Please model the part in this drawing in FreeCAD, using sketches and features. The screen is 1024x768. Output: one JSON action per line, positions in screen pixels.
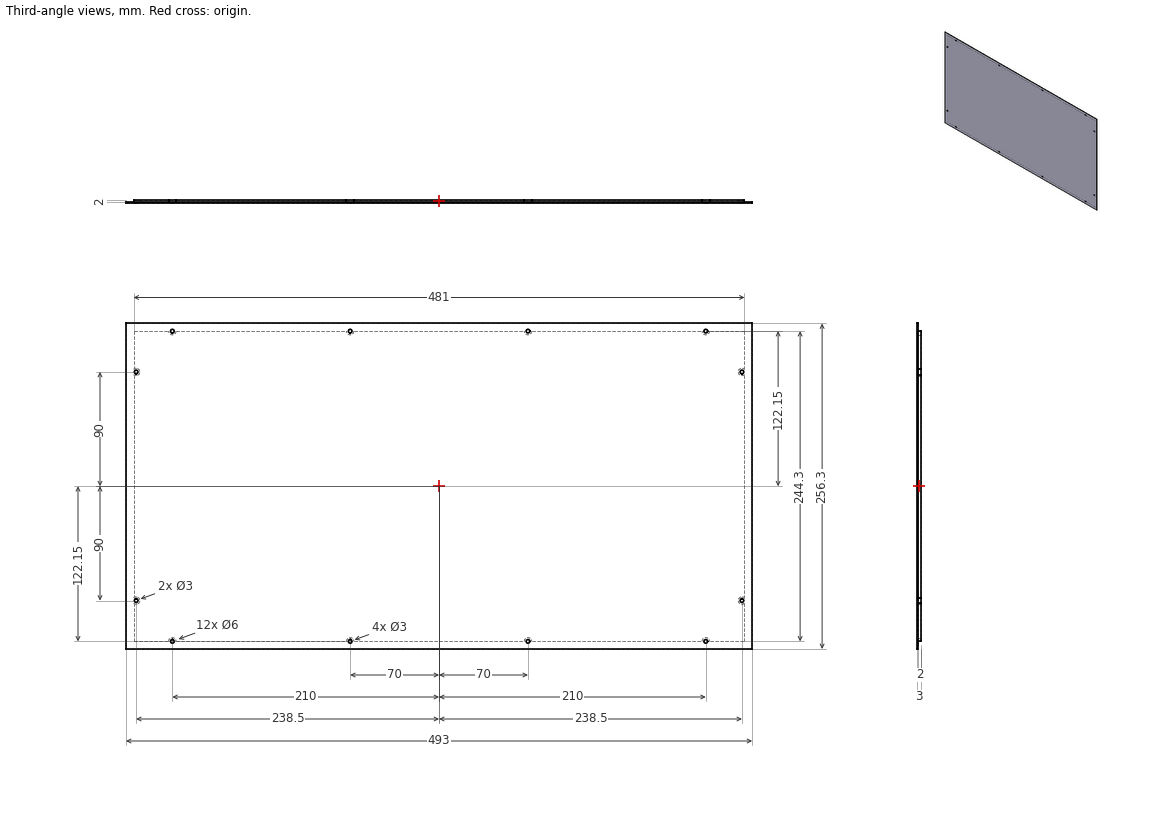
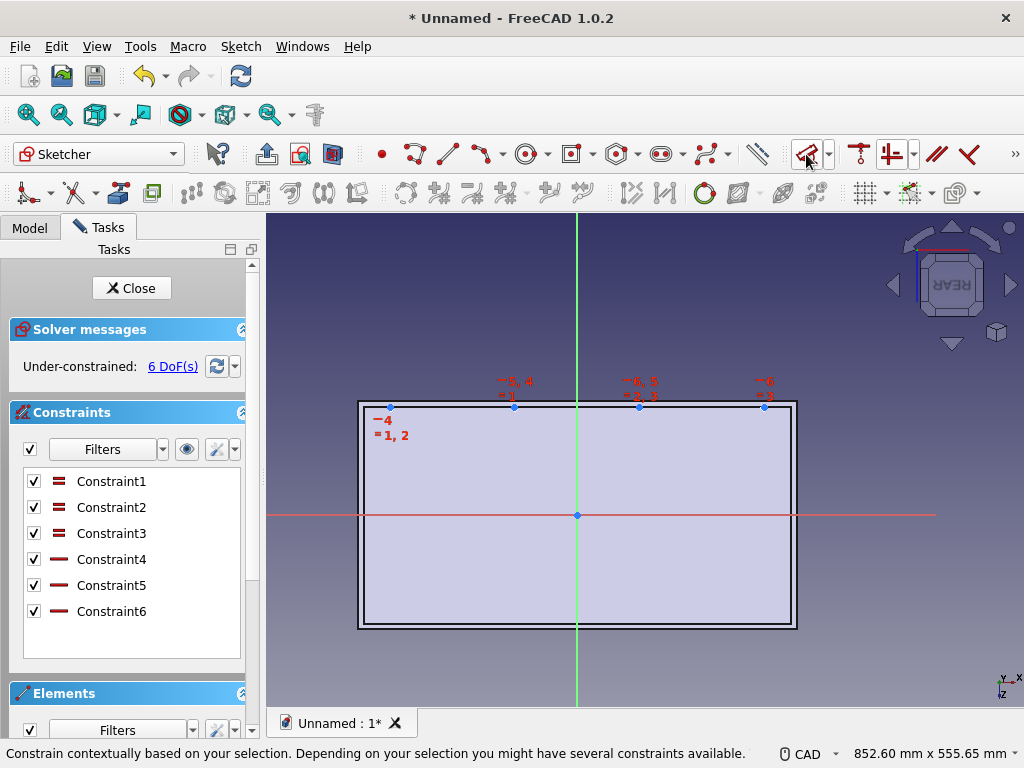
{"action": "scroll", "coordinate": [517, 406], "scroll_direction": "up", "scroll_amount": 14}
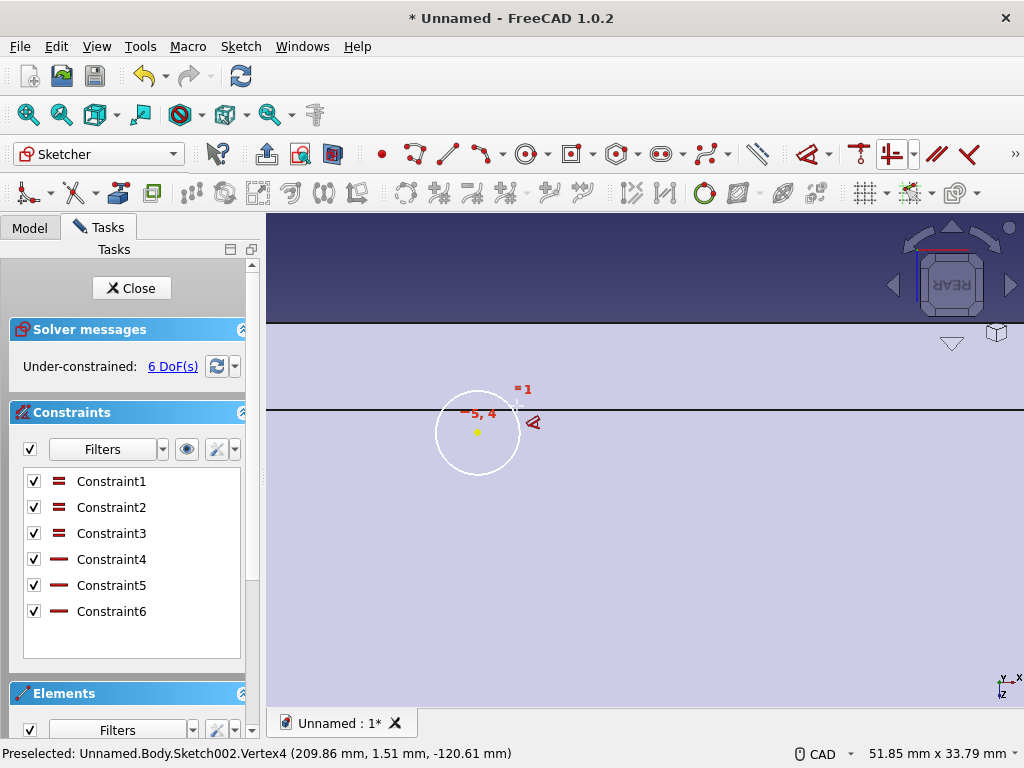
{"action": "left_click", "coordinate": [507, 403]}
{"action": "left_click", "coordinate": [529, 380]}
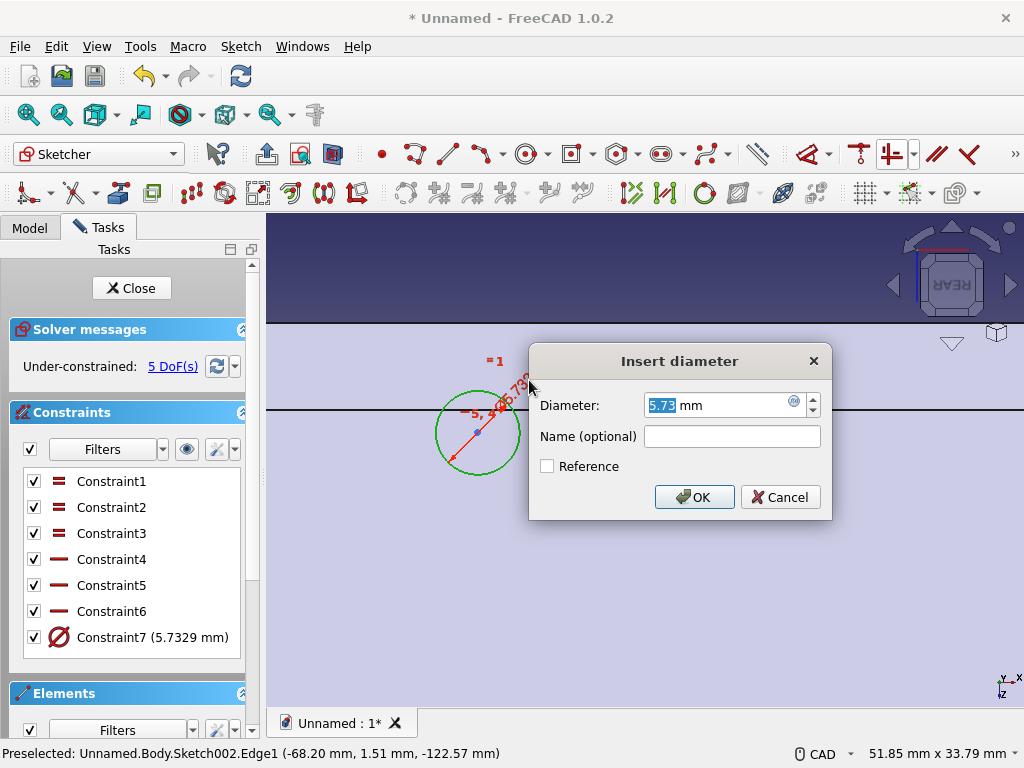
{"action": "type", "text": "3"}
{"action": "key", "text": "Return"}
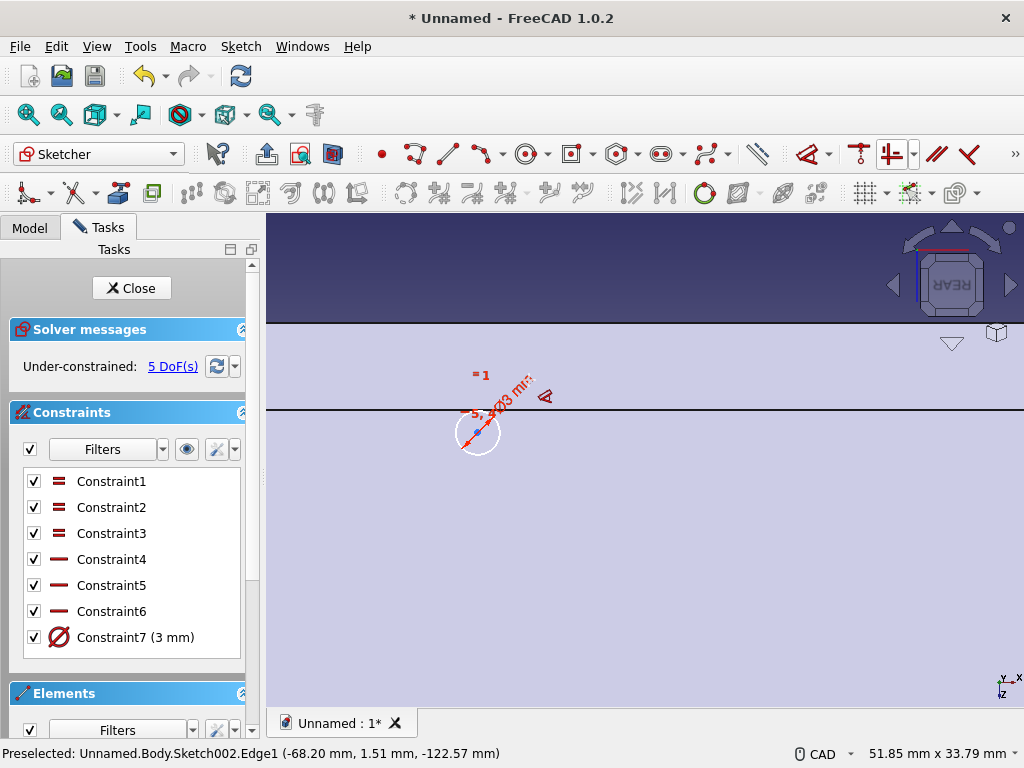
{"action": "scroll", "coordinate": [516, 406], "scroll_direction": "down", "scroll_amount": 14}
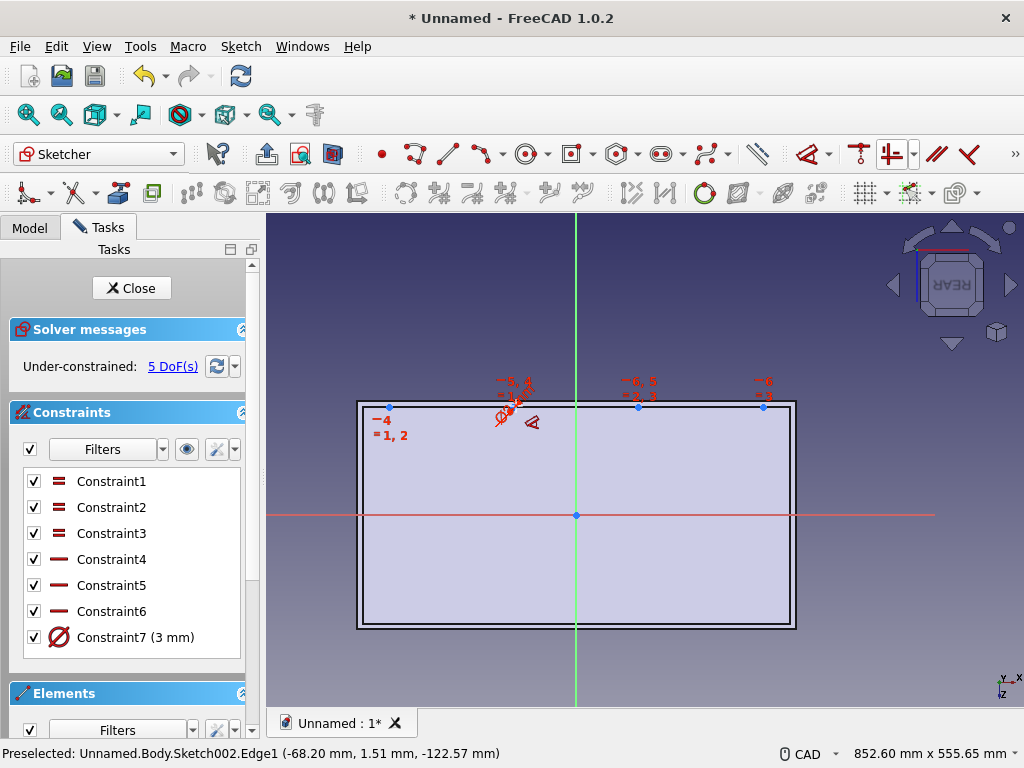
{"action": "left_click", "coordinate": [514, 408]}
{"action": "left_click", "coordinate": [545, 549]}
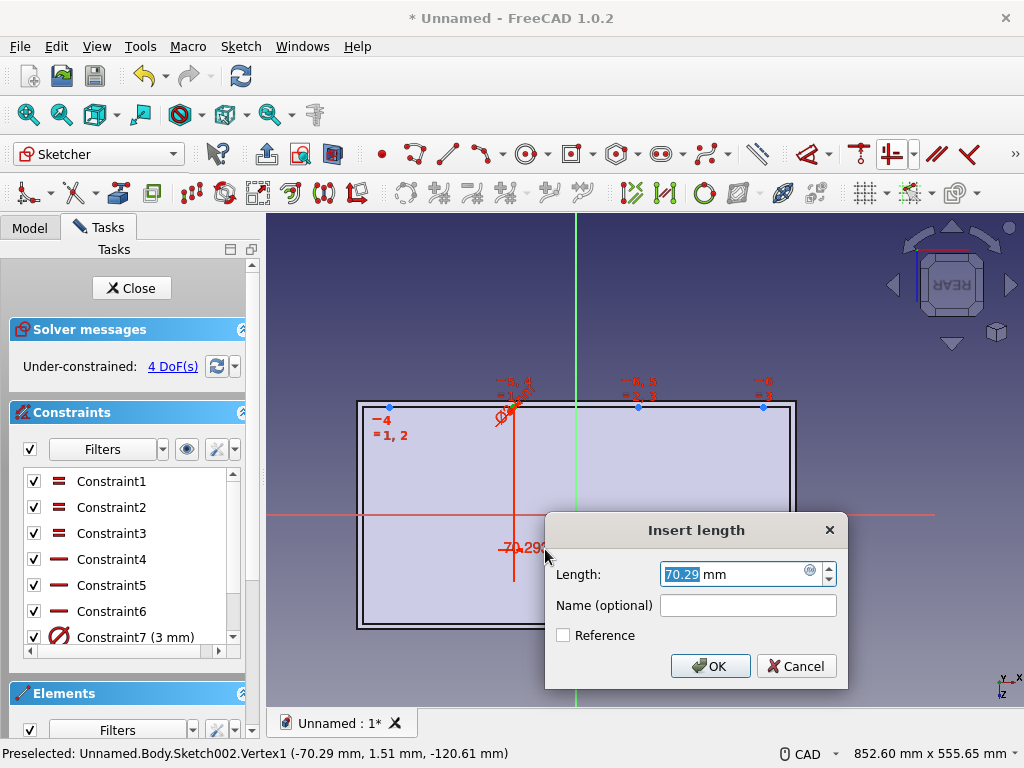
{"action": "type", "text": "70"}
{"action": "key", "text": "Return"}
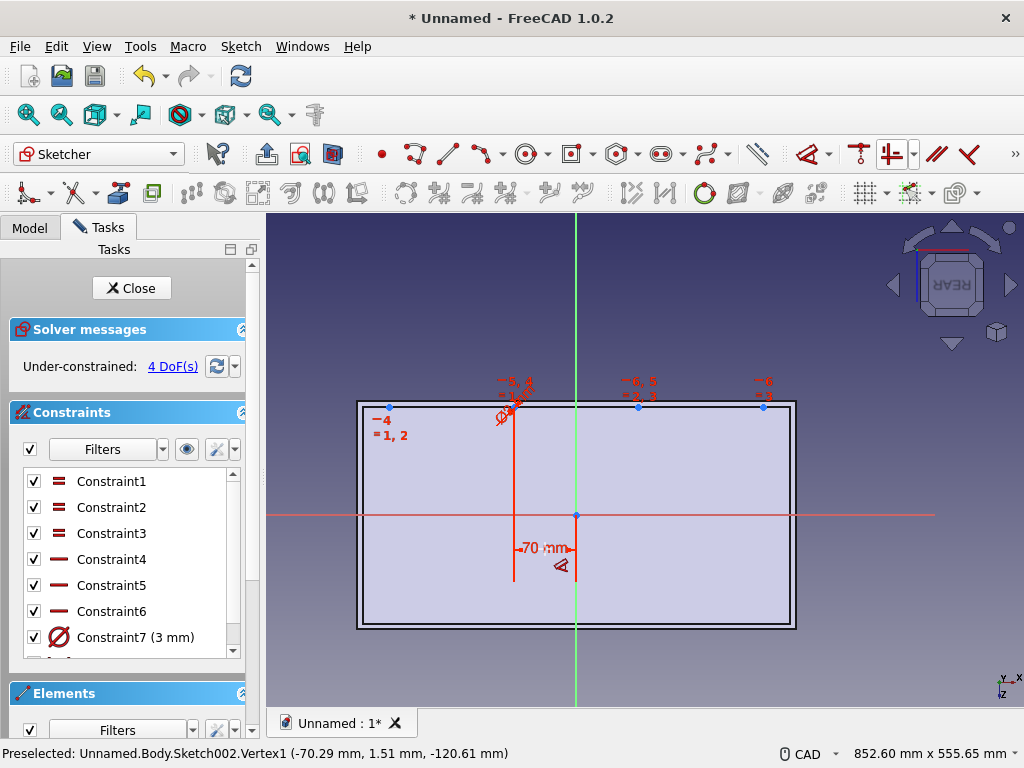
{"action": "left_click", "coordinate": [639, 408]}
{"action": "left_click", "coordinate": [622, 549]}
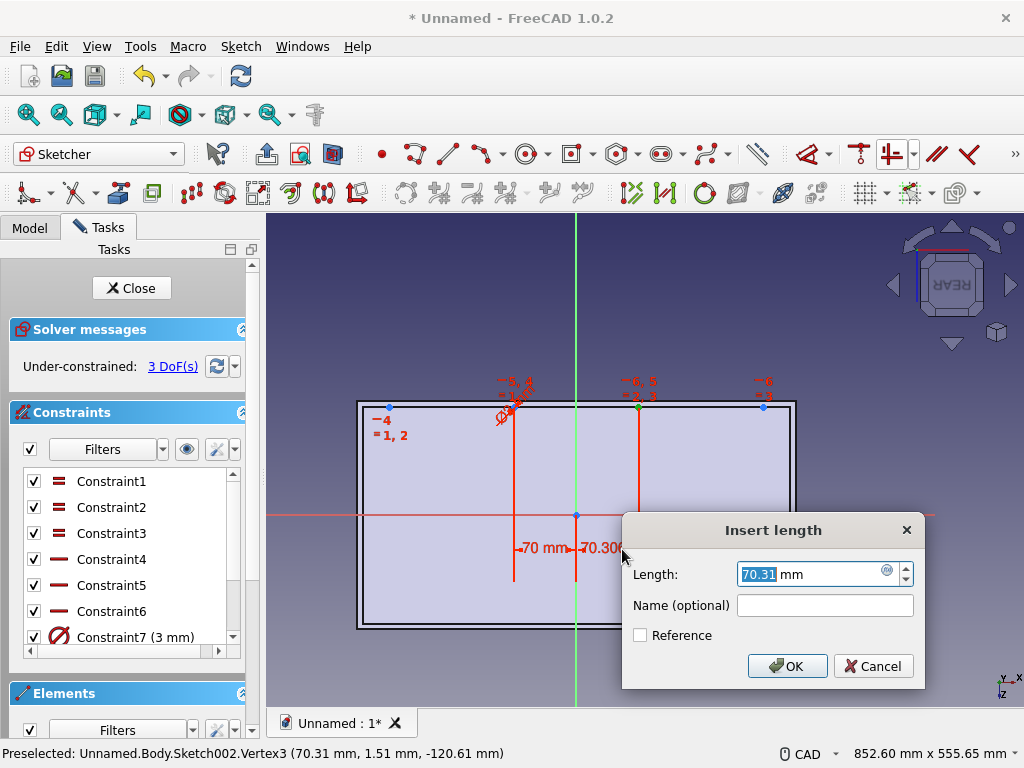
{"action": "type", "text": "70"}
{"action": "key", "text": "Return"}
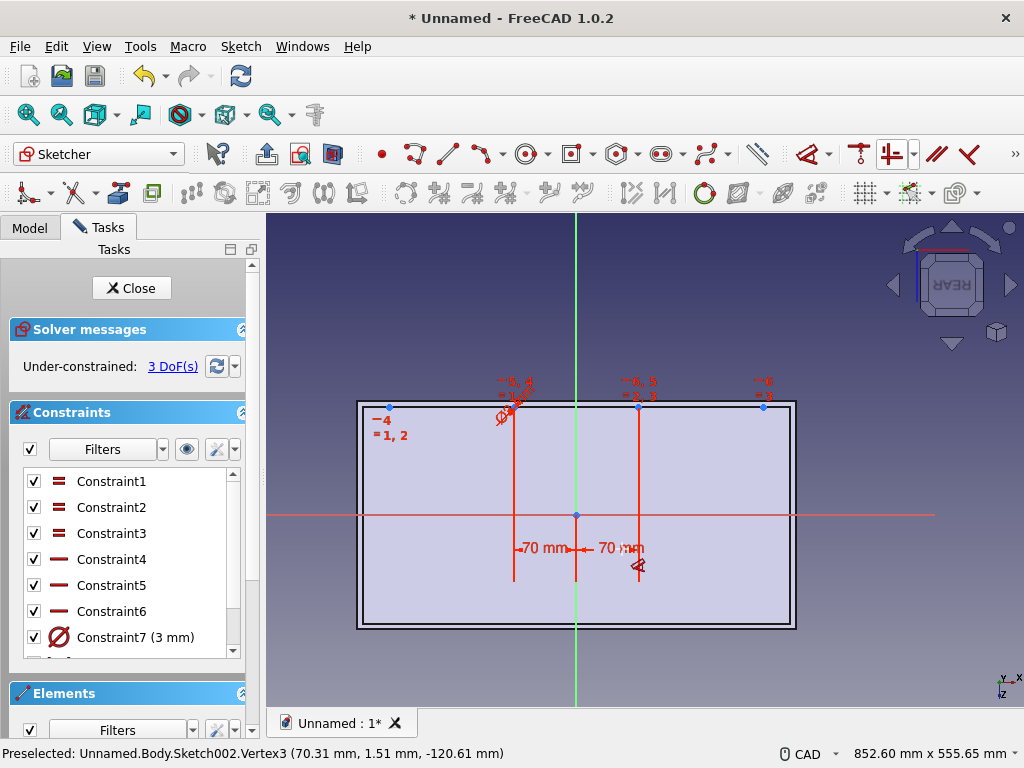
{"action": "left_click", "coordinate": [390, 408]}
{"action": "left_click", "coordinate": [440, 549]}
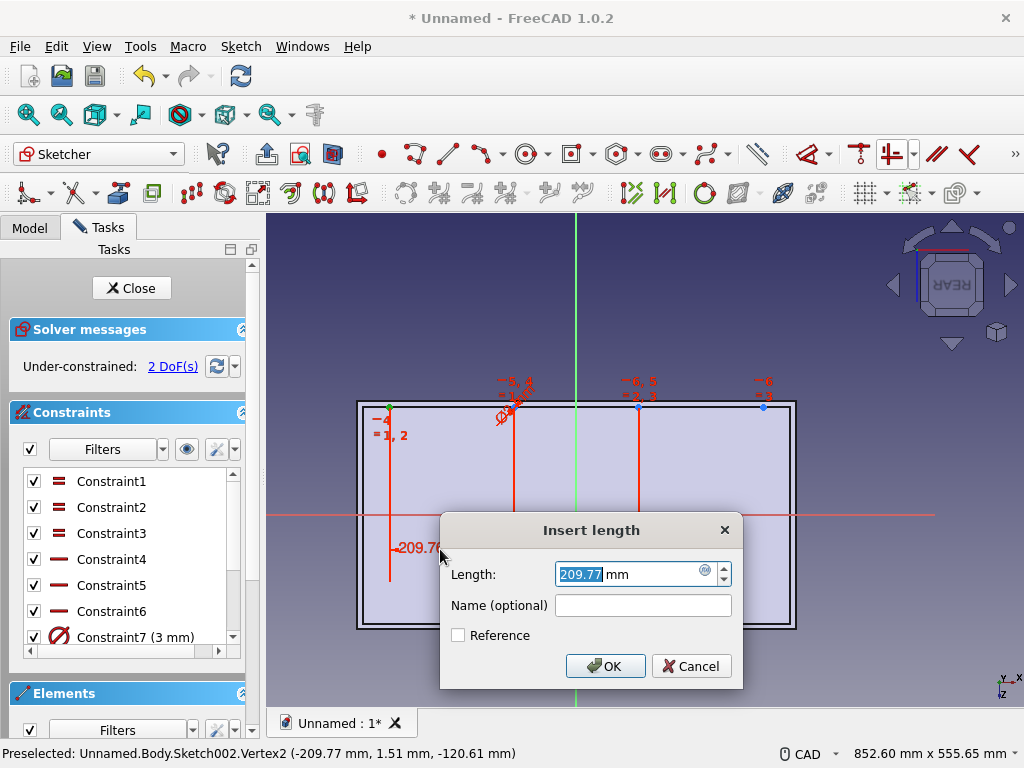
{"action": "type", "text": "210"}
{"action": "key", "text": "Return"}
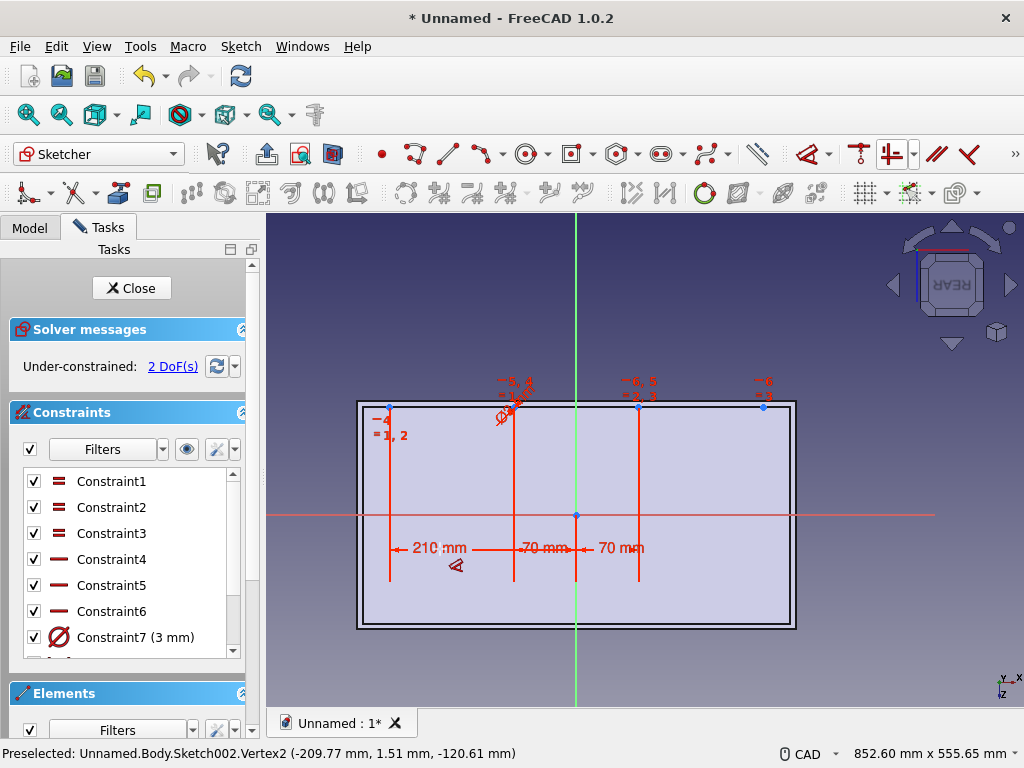
{"action": "left_click", "coordinate": [763, 408]}
{"action": "left_click", "coordinate": [713, 549]}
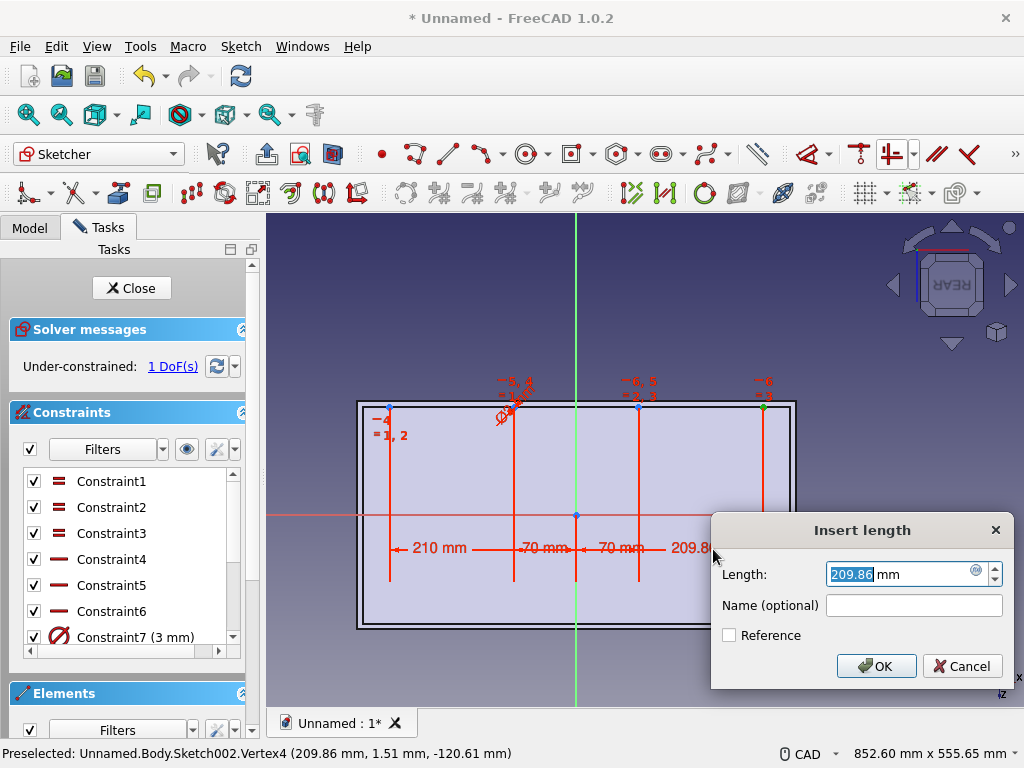
{"action": "type", "text": "210"}
{"action": "key", "text": "Return"}